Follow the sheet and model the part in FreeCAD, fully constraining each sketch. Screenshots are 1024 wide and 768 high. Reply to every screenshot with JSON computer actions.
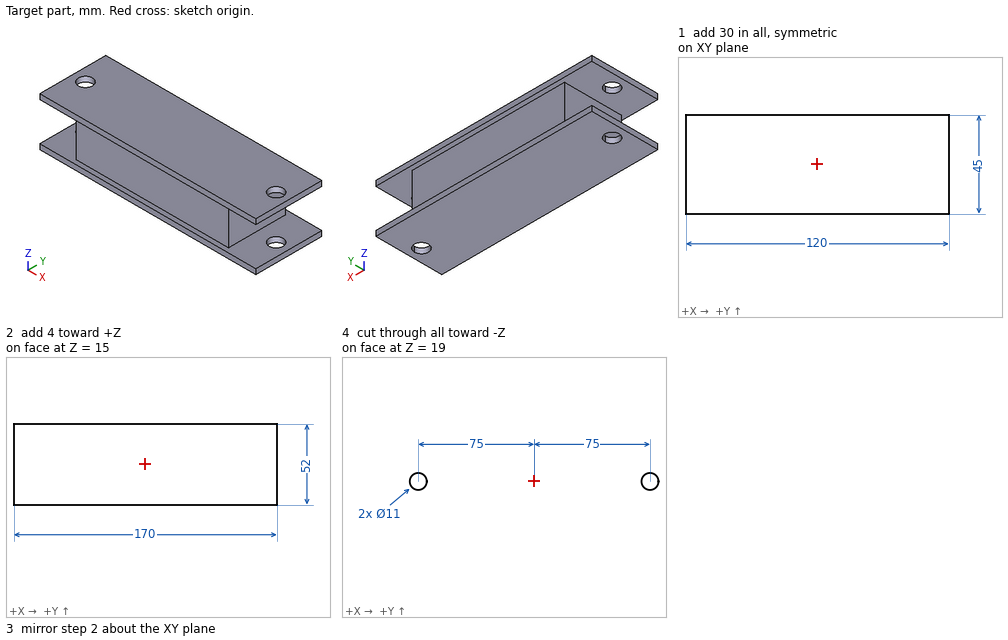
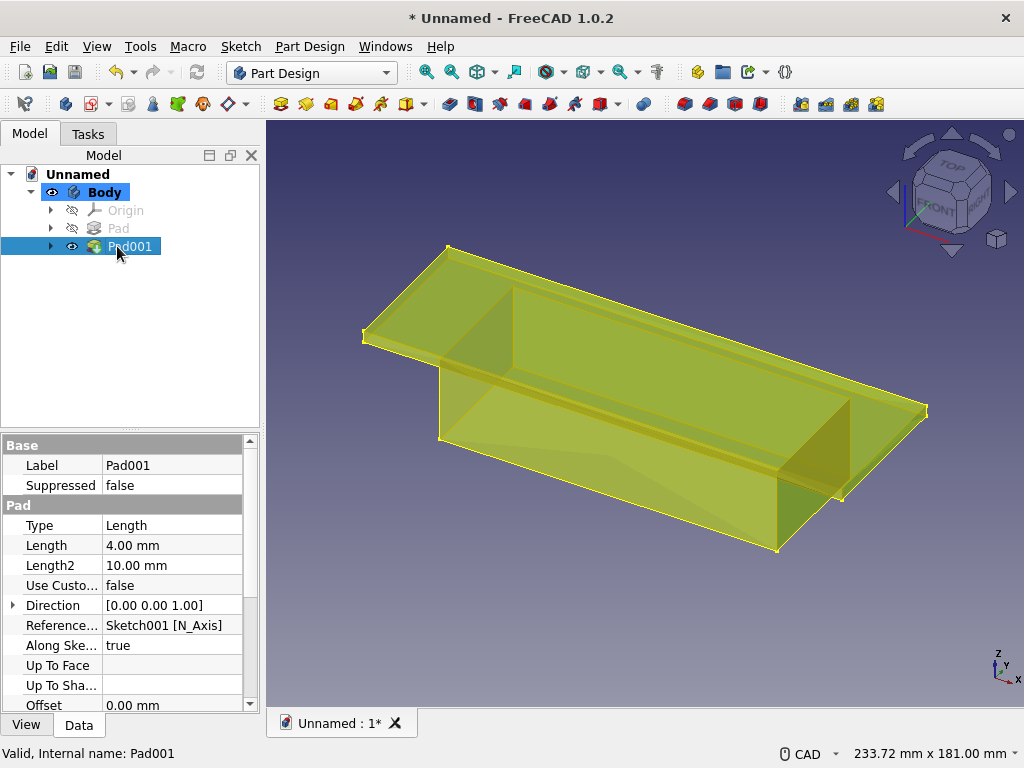
{"action": "left_click", "coordinate": [801, 104]}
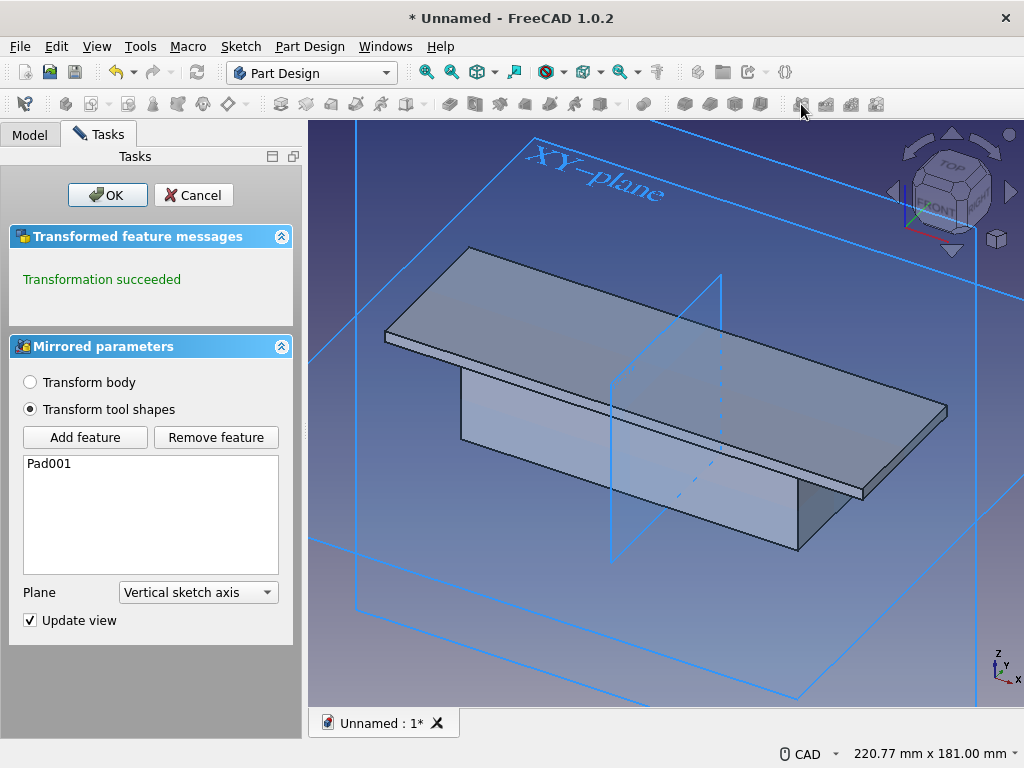
{"action": "left_click", "coordinate": [199, 592]}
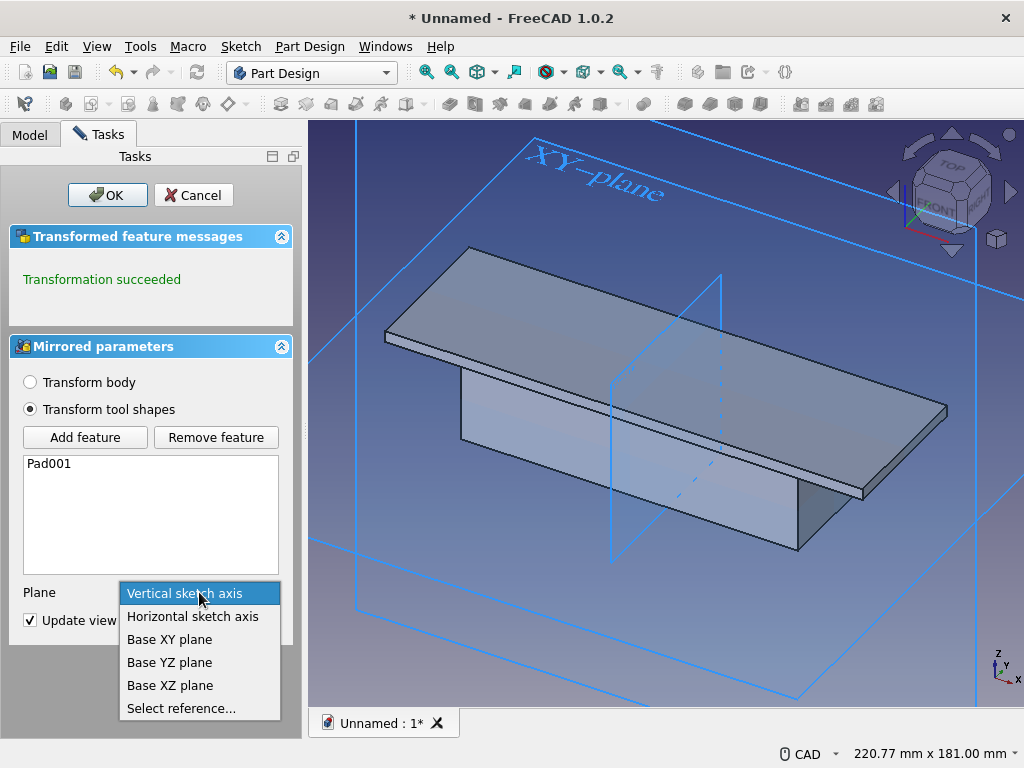
{"action": "left_click", "coordinate": [198, 640]}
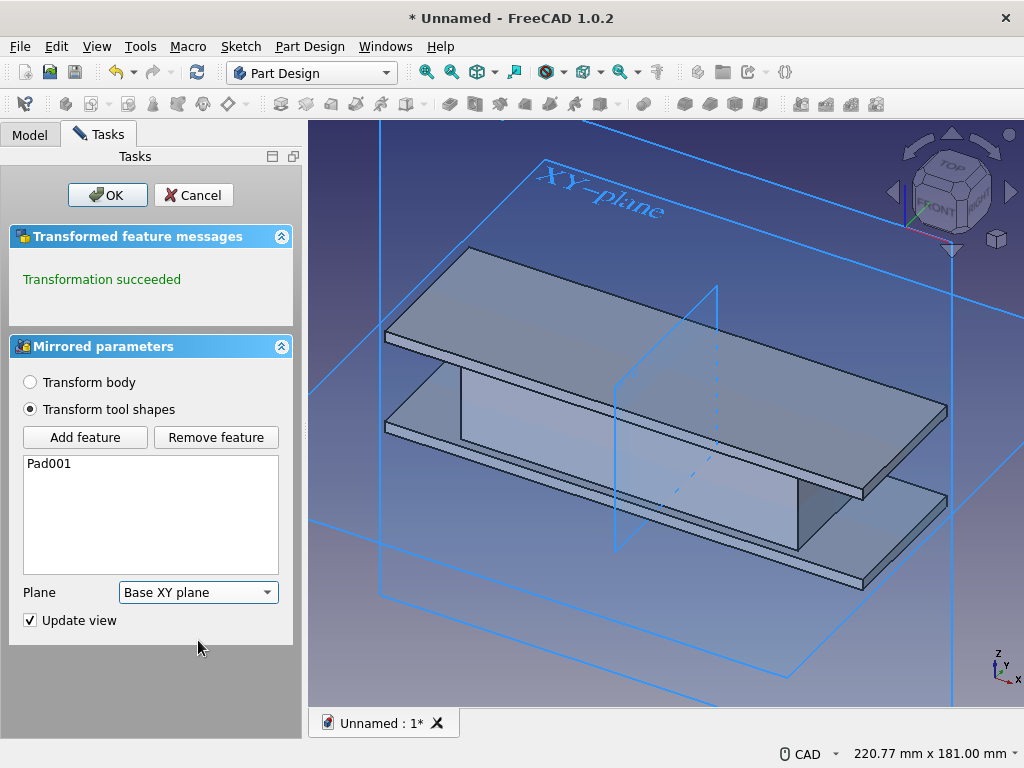
{"action": "left_click", "coordinate": [108, 195]}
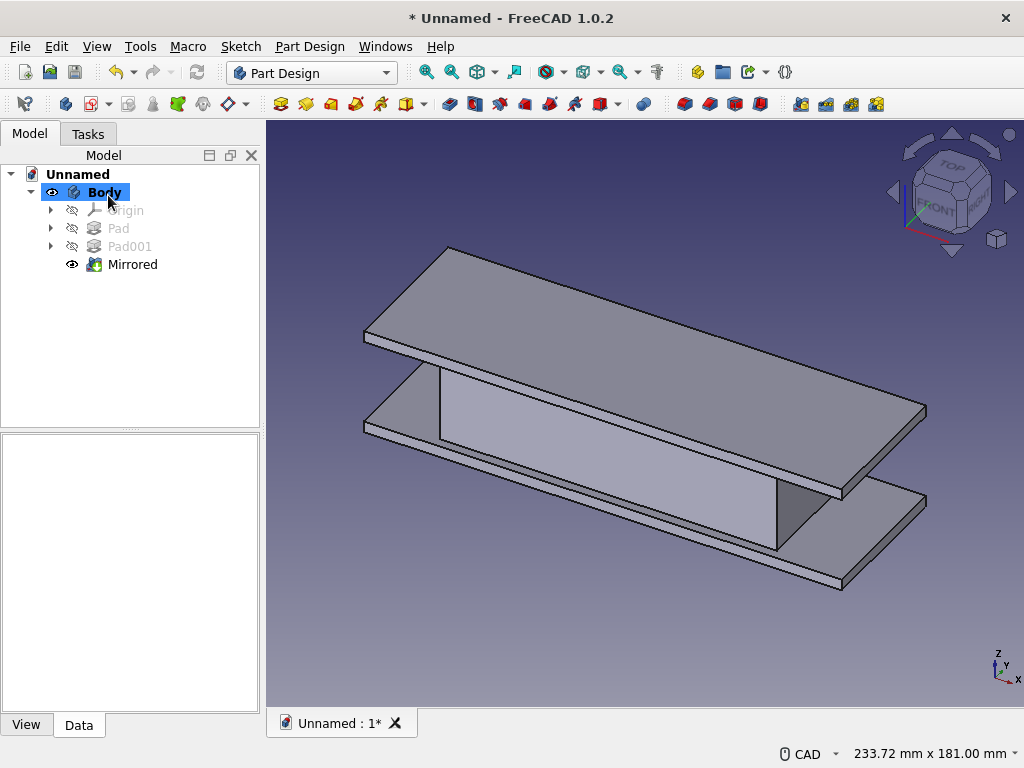
{"action": "left_click", "coordinate": [781, 413]}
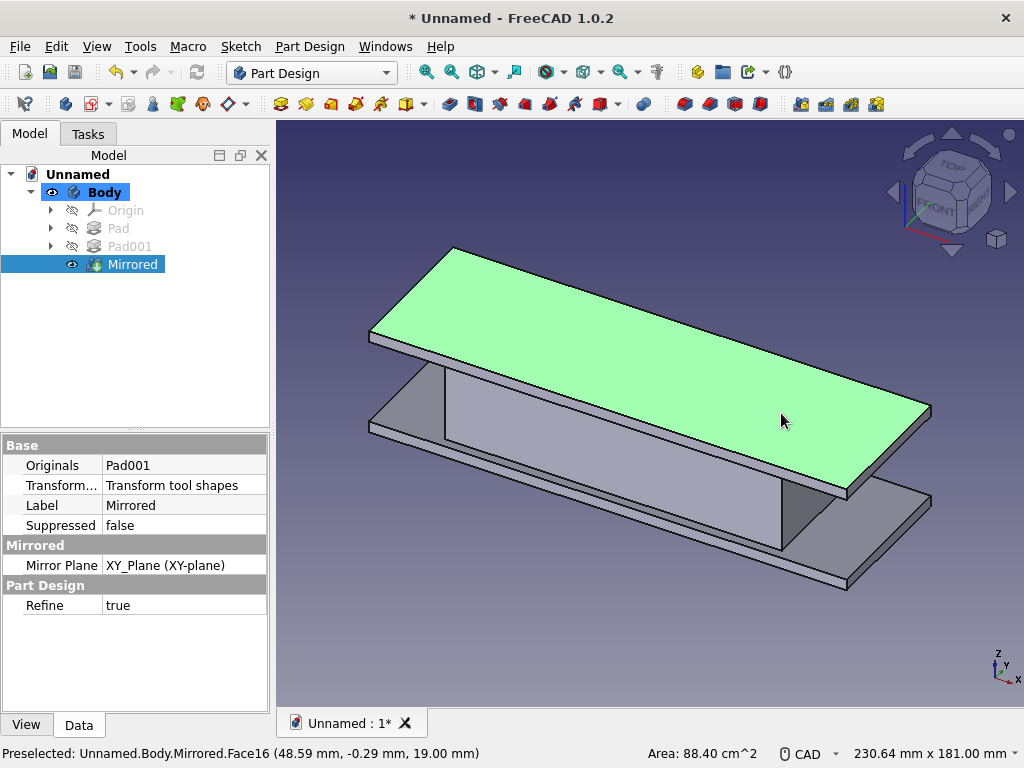
{"action": "left_click", "coordinate": [90, 104]}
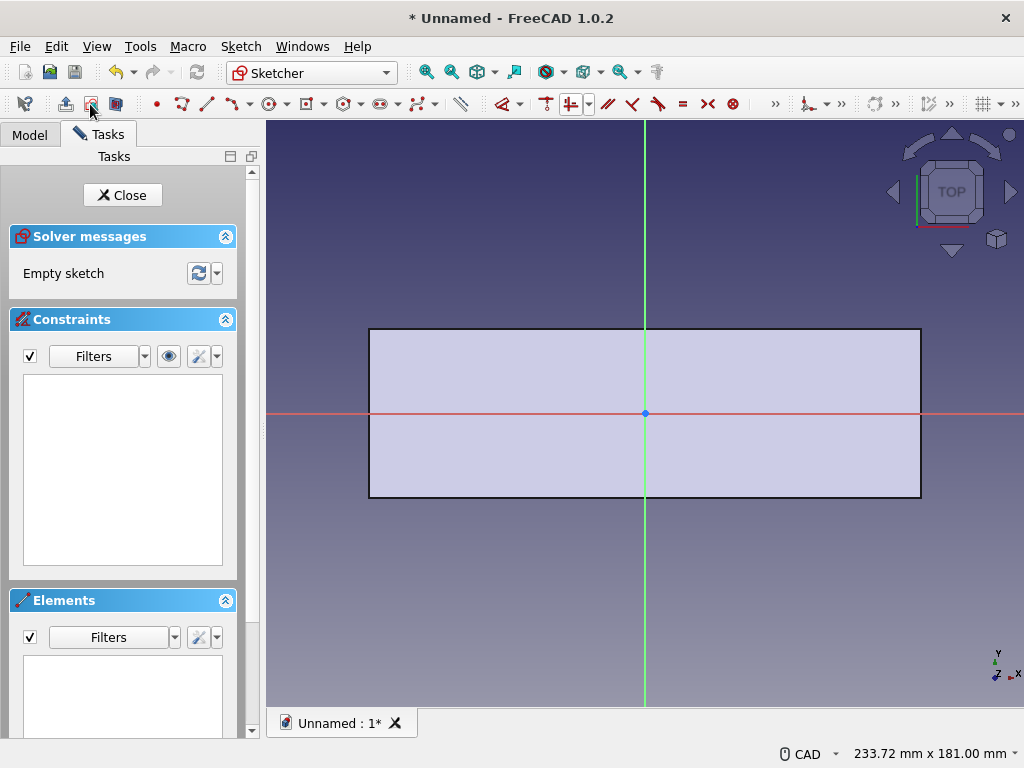
{"action": "scroll", "coordinate": [294, 413], "scroll_direction": "down", "scroll_amount": 1}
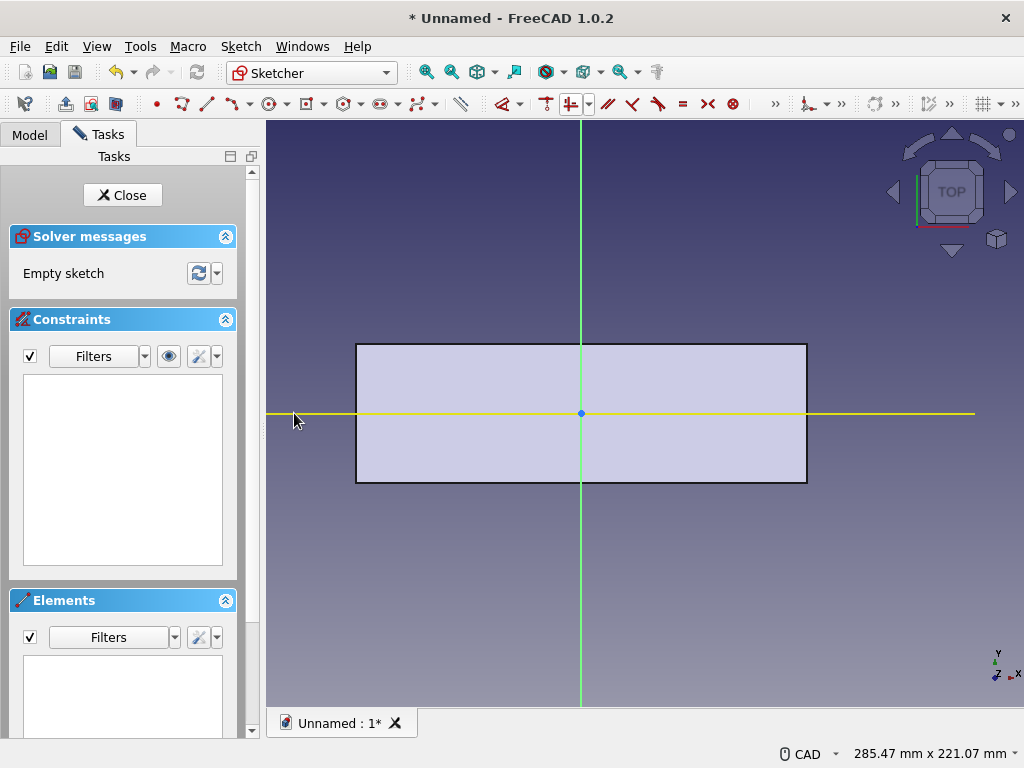
{"action": "left_click", "coordinate": [268, 104]}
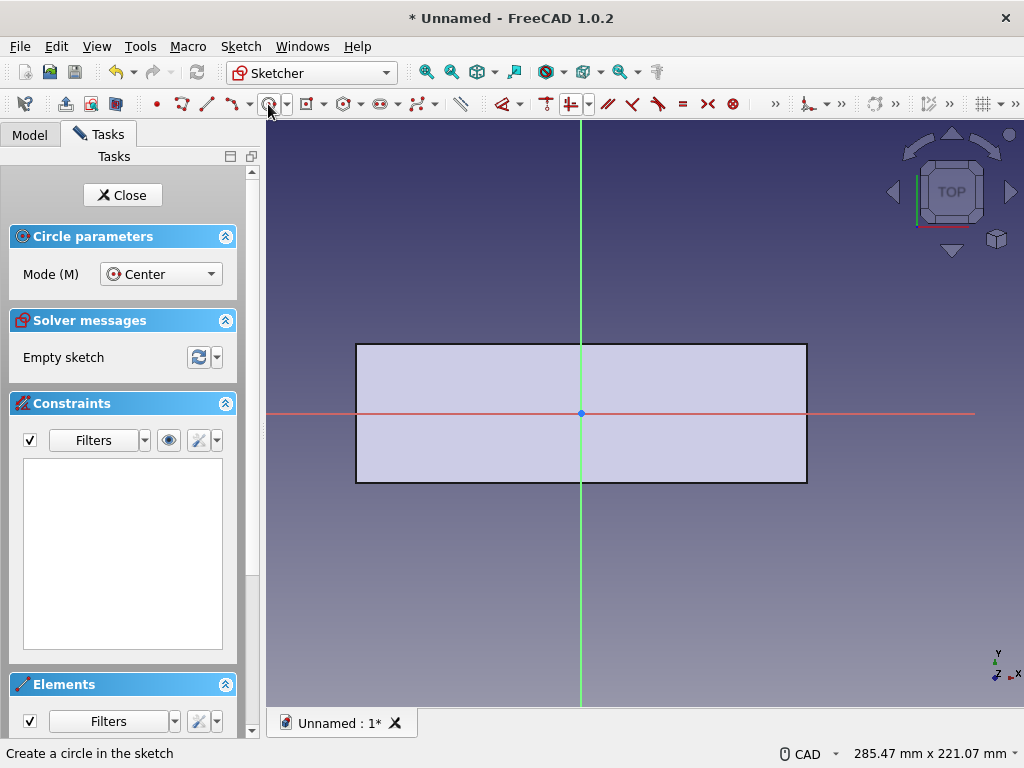
{"action": "scroll", "coordinate": [382, 414], "scroll_direction": "up", "scroll_amount": 3}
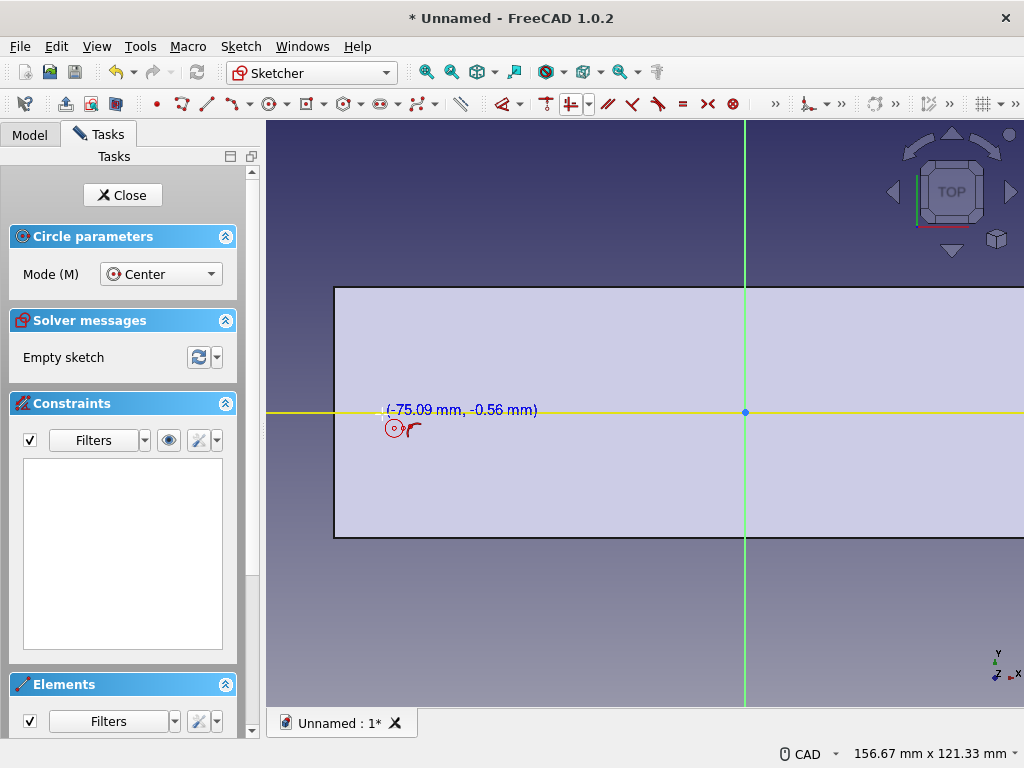
{"action": "left_click", "coordinate": [382, 413]}
{"action": "mouse_move", "coordinate": [401, 394]}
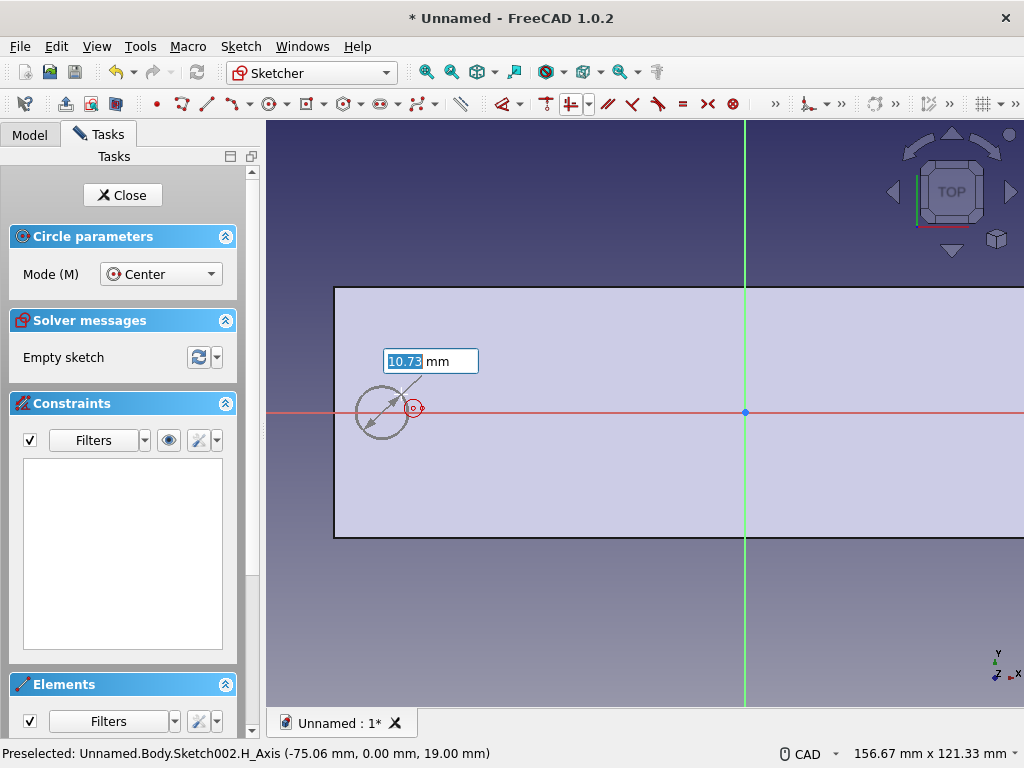
{"action": "type", "text": "11"}
{"action": "key", "text": "Return"}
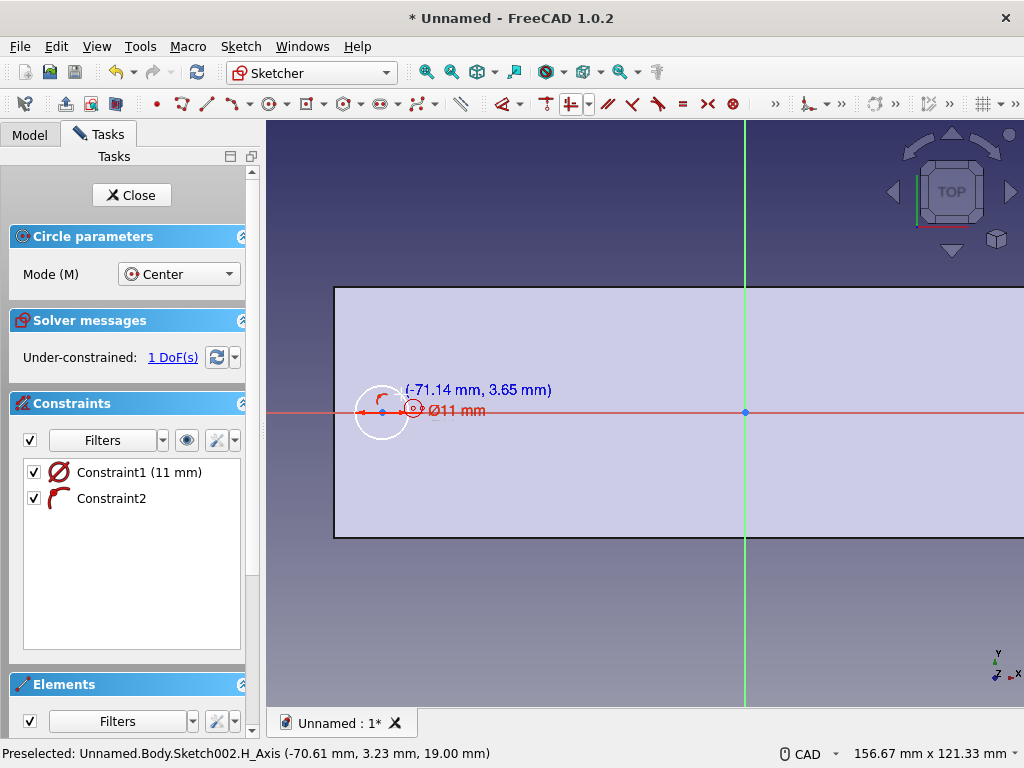
{"action": "scroll", "coordinate": [371, 415], "scroll_direction": "down", "scroll_amount": 3}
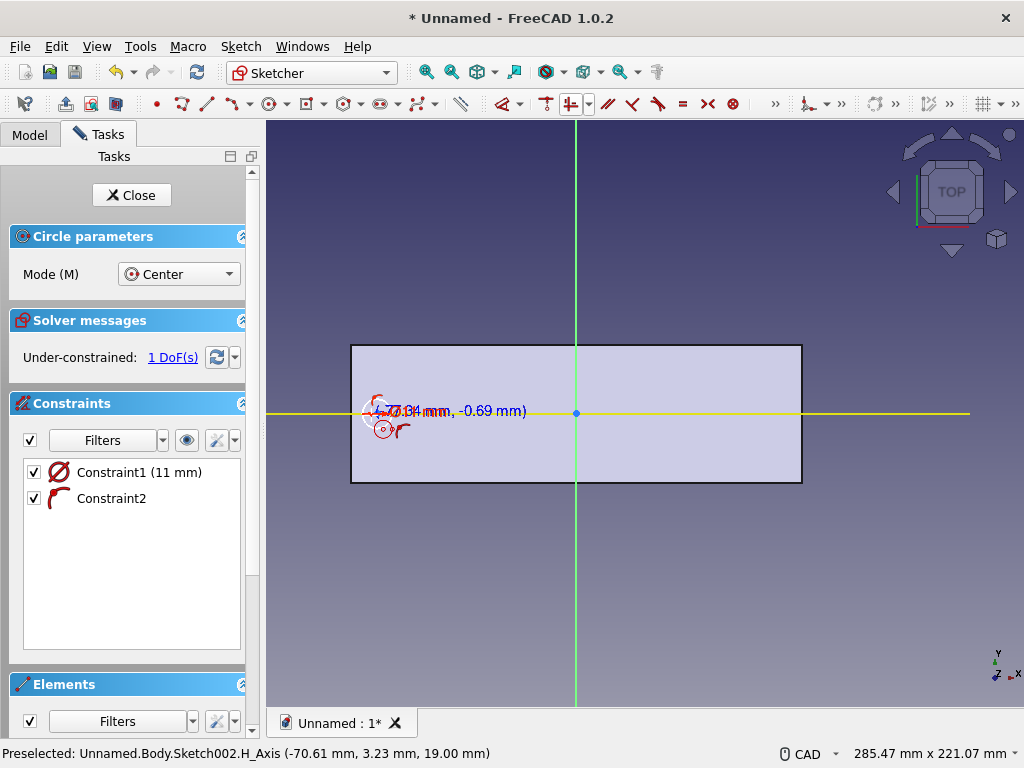
{"action": "scroll", "coordinate": [776, 414], "scroll_direction": "up", "scroll_amount": 3}